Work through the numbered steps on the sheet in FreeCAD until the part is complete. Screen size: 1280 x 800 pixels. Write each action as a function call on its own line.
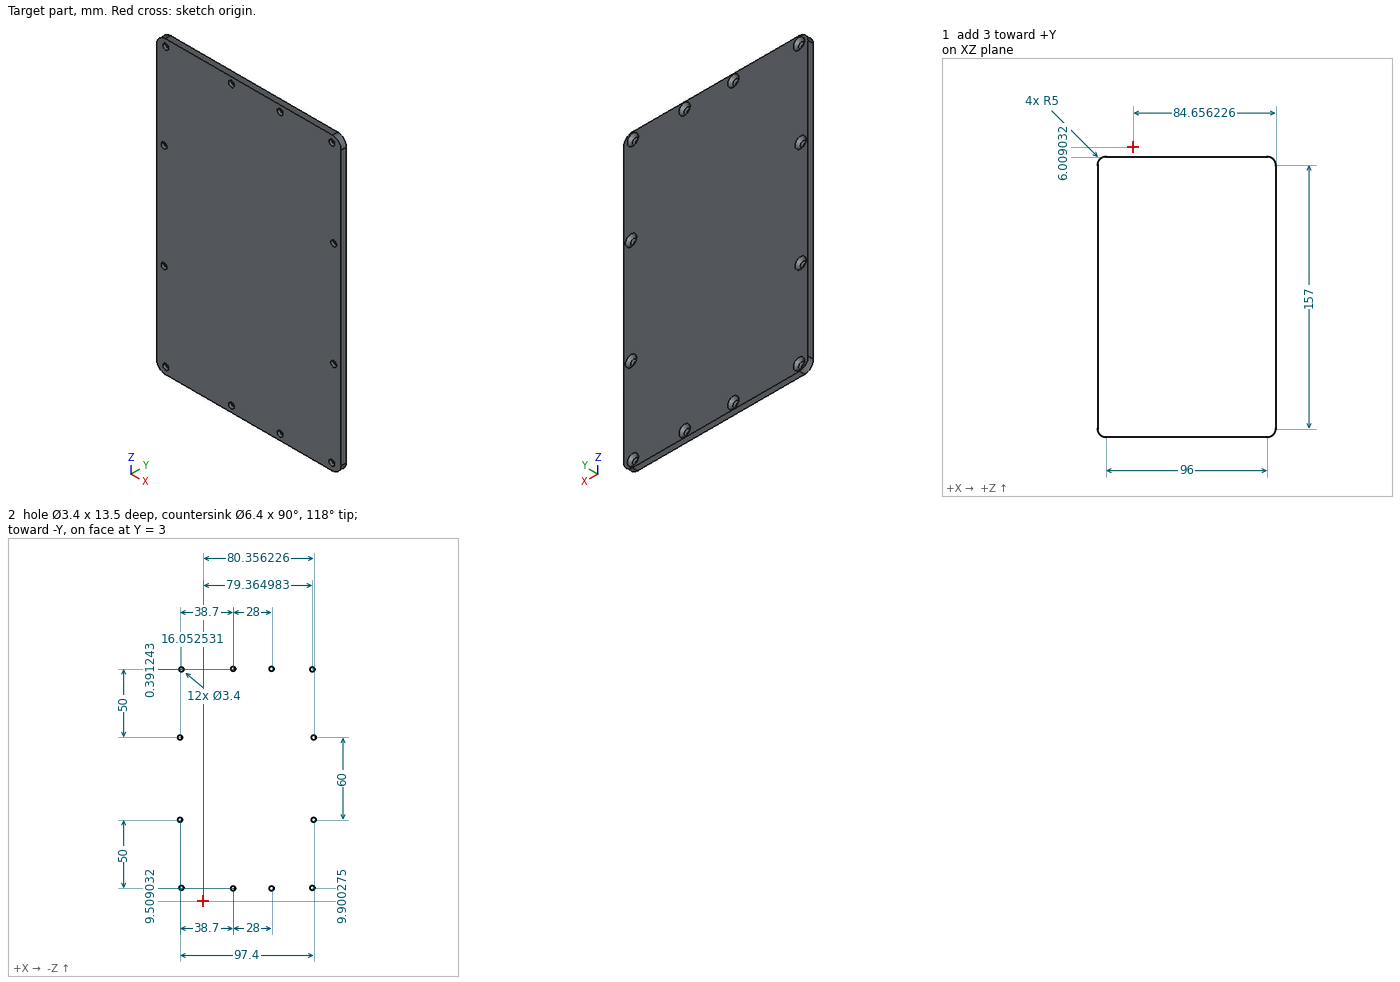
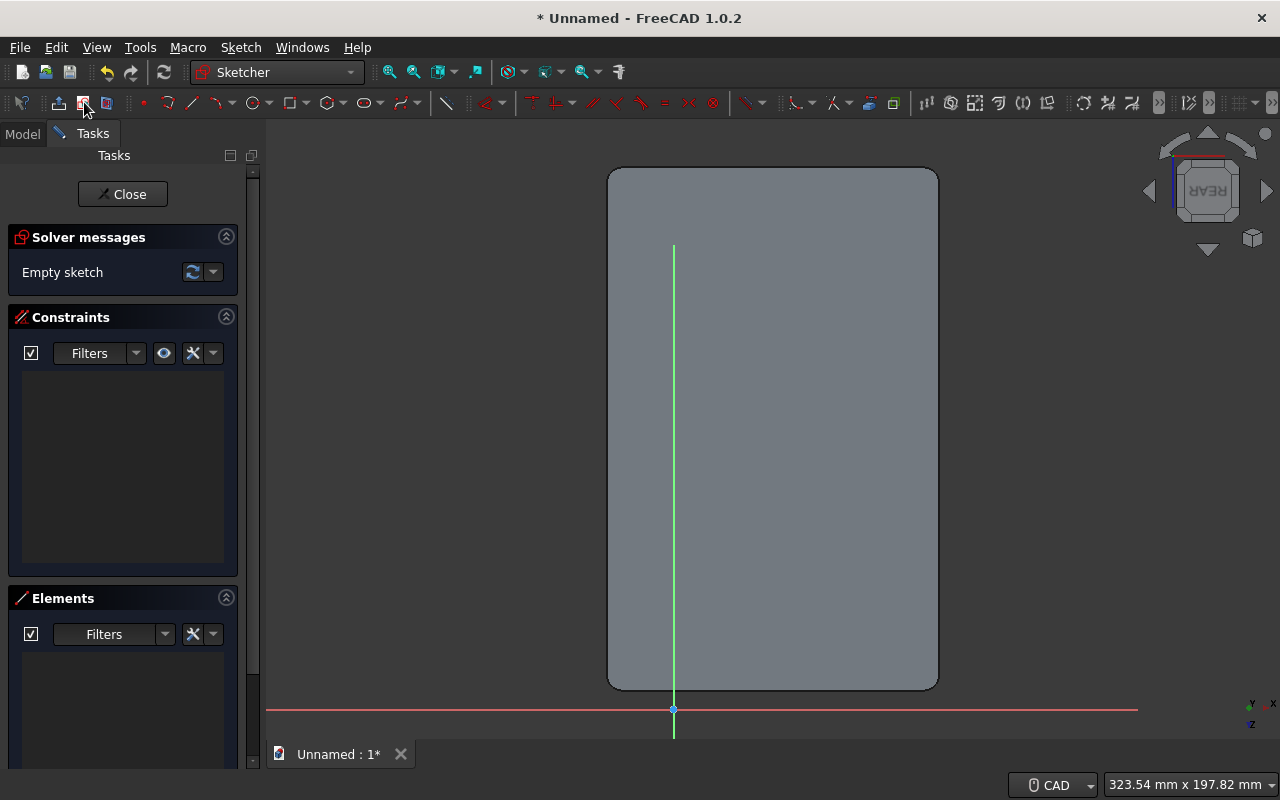
scroll(395, 374, down, 1)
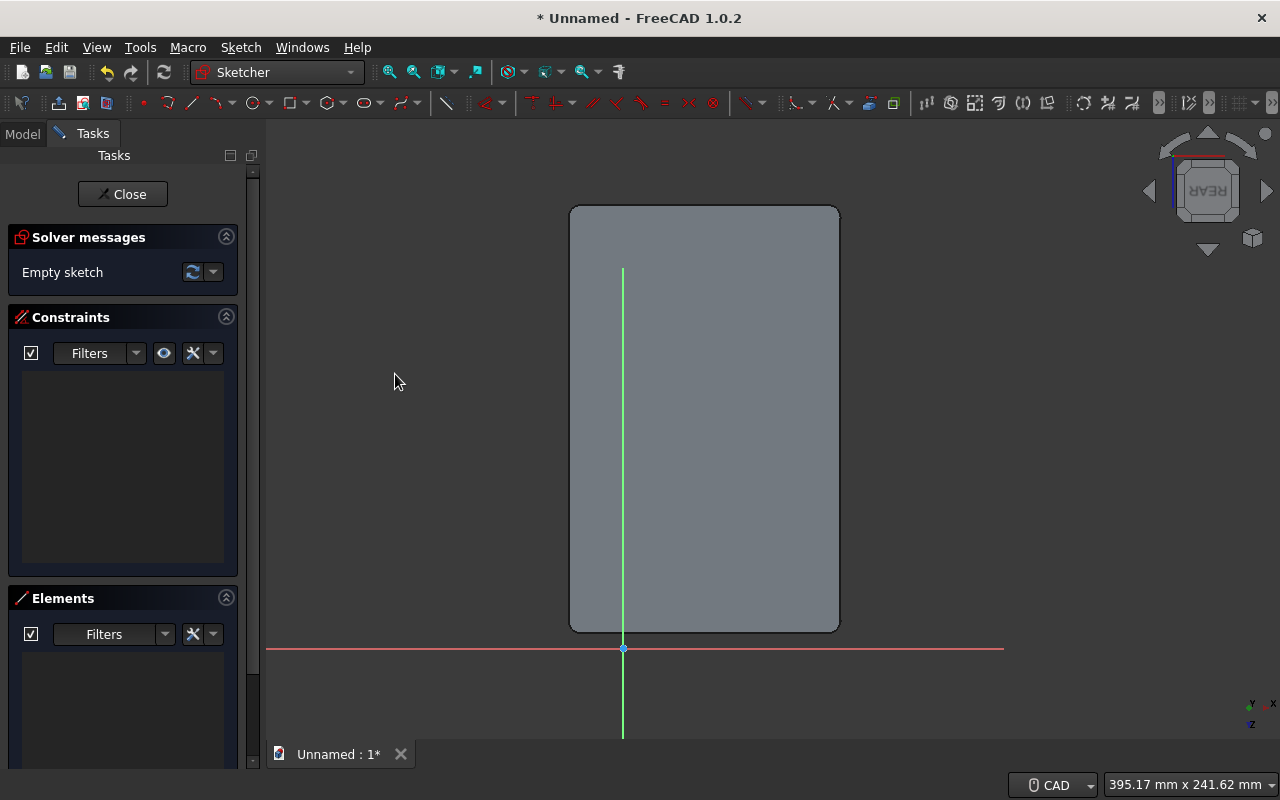
click(254, 104)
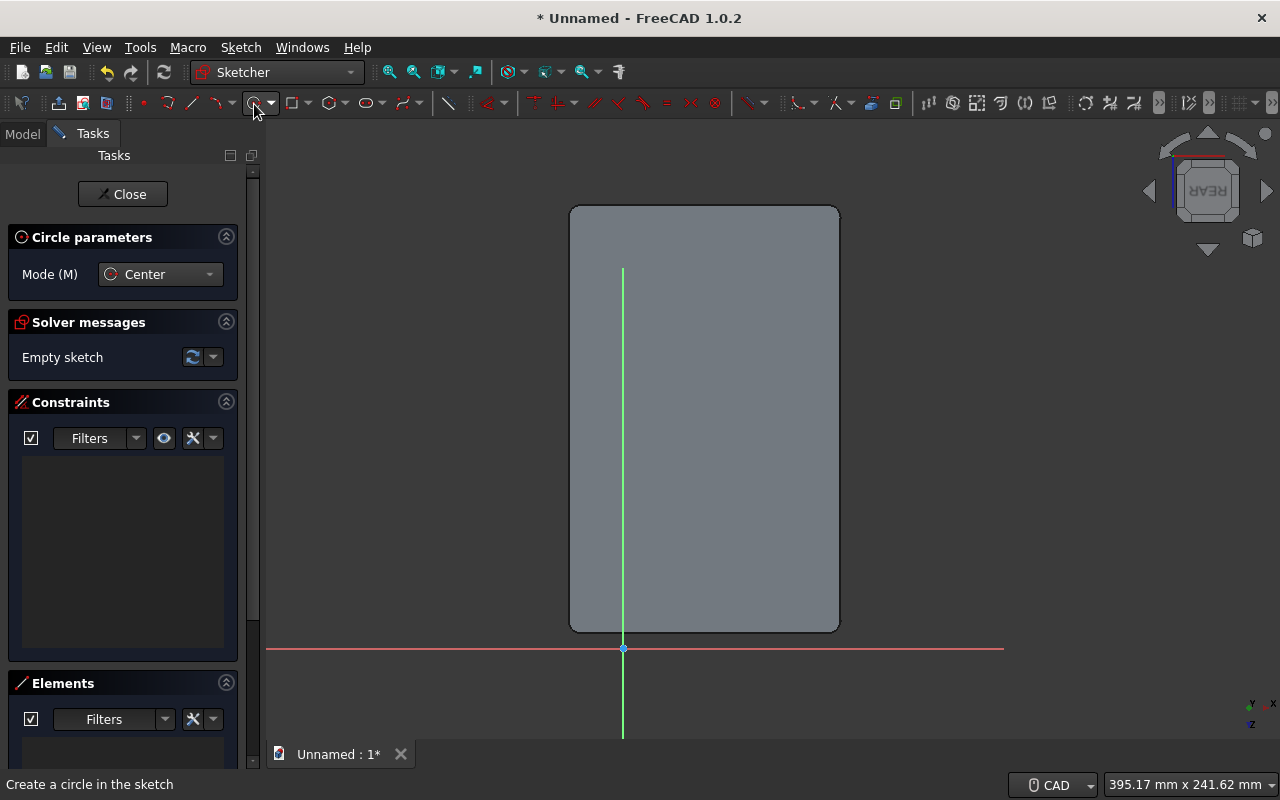
scroll(582, 215, up, 9)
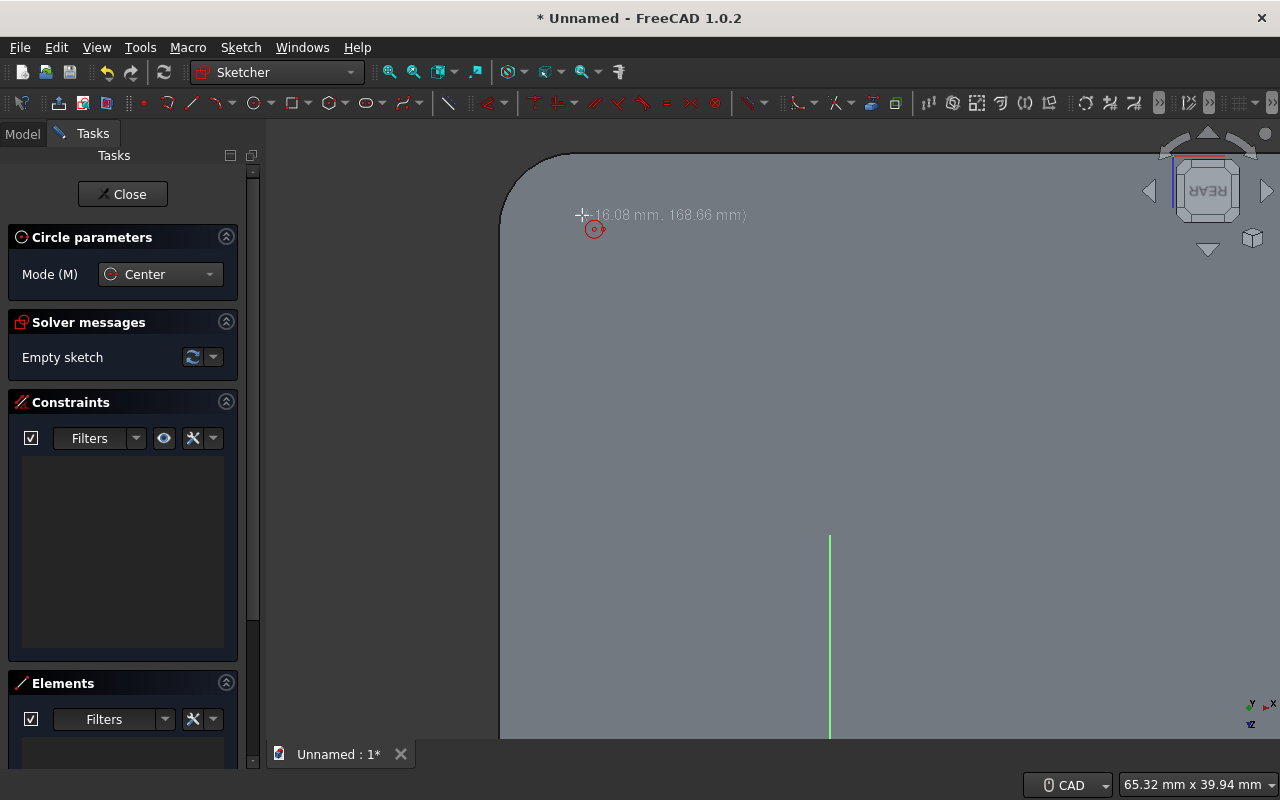
scroll(582, 215, down, 9)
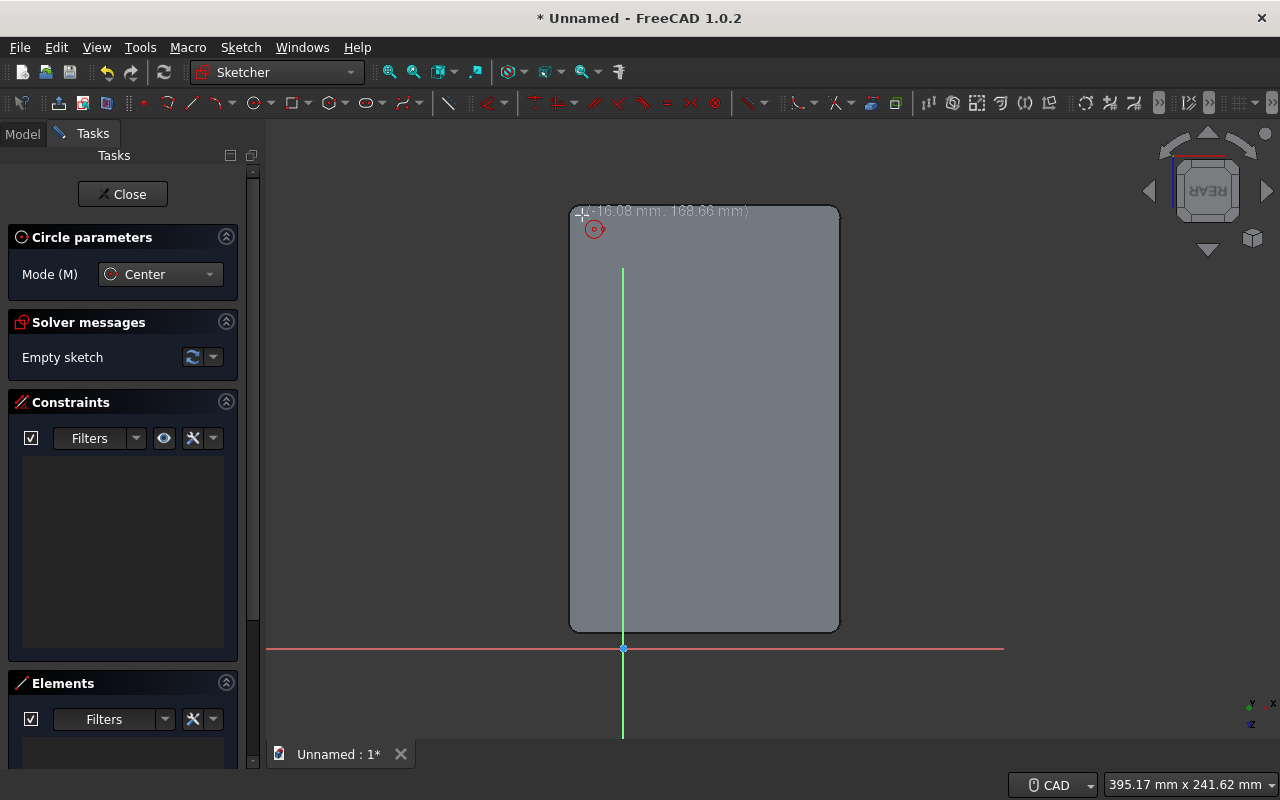
click(582, 215)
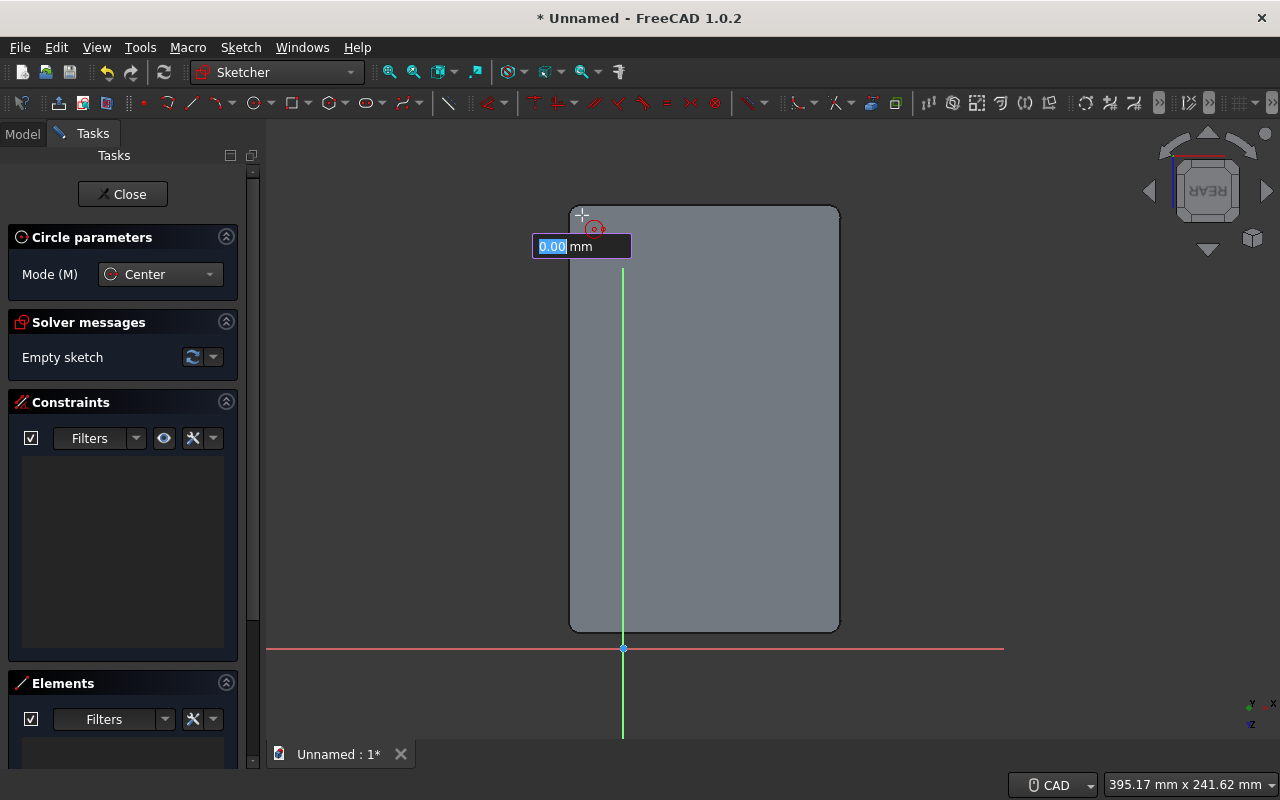
scroll(585, 212, up, 7)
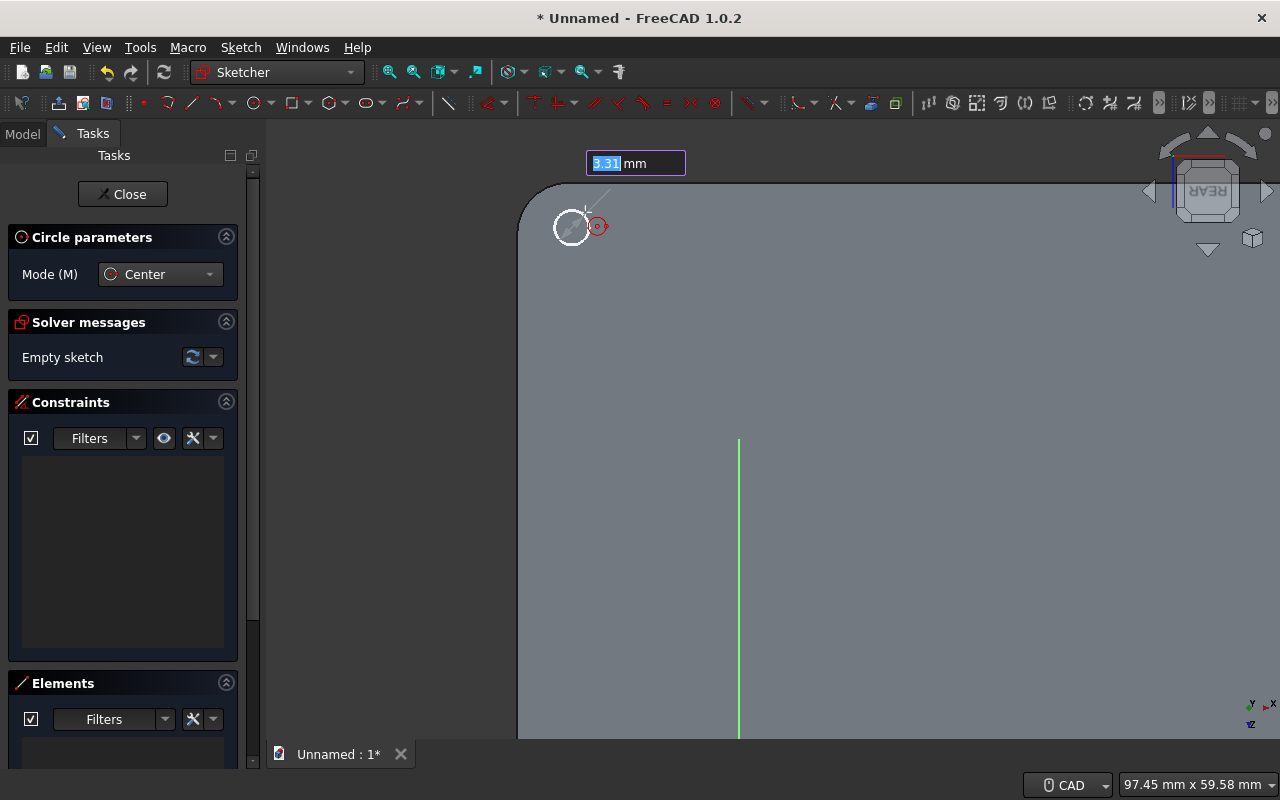
click(585, 211)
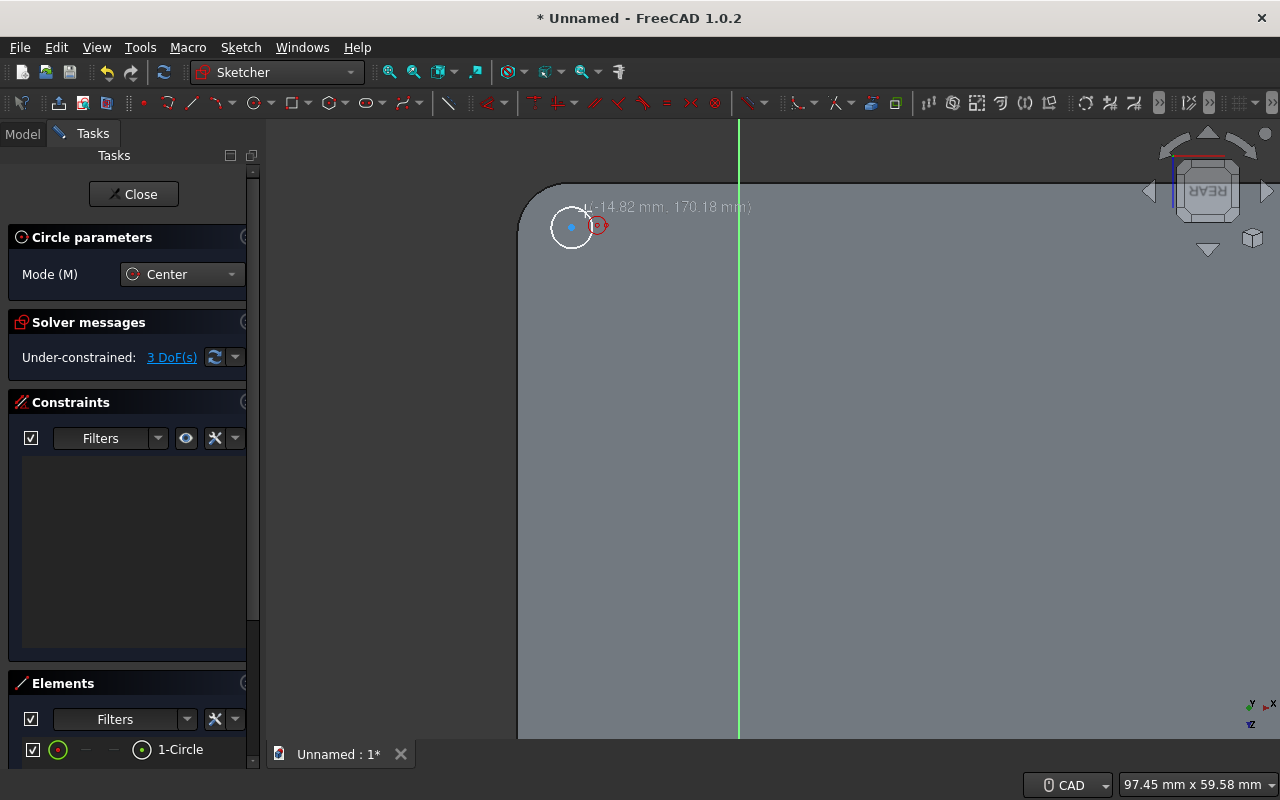
scroll(585, 212, down, 7)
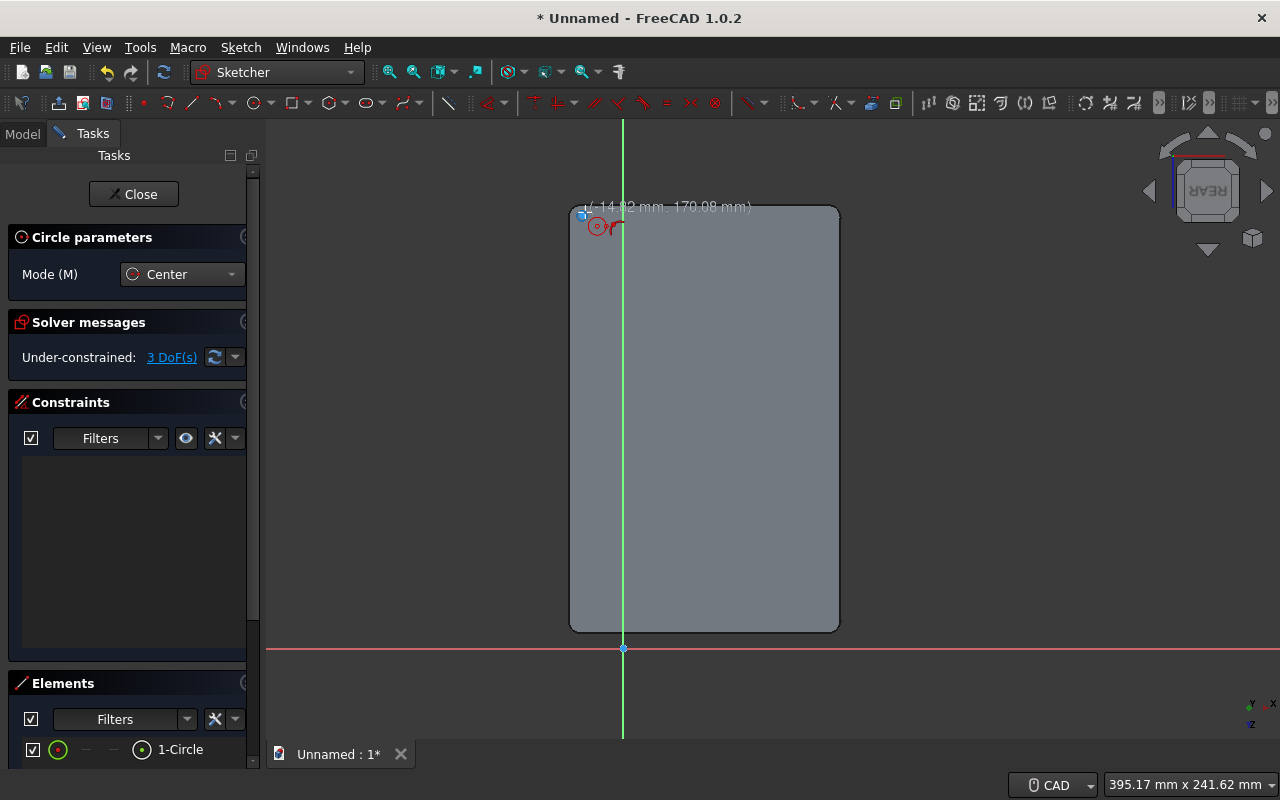
scroll(827, 215, up, 9)